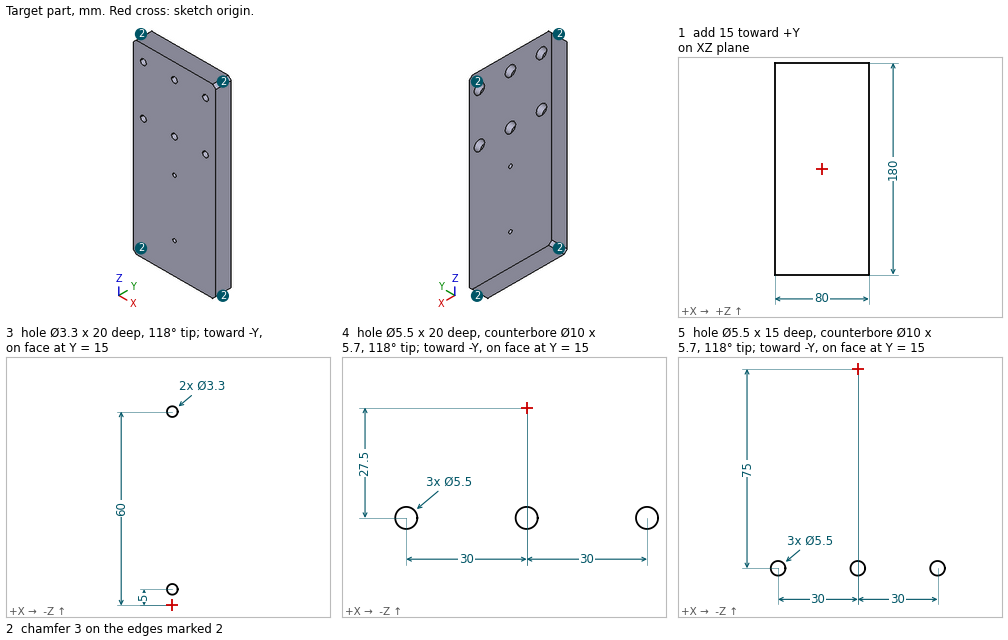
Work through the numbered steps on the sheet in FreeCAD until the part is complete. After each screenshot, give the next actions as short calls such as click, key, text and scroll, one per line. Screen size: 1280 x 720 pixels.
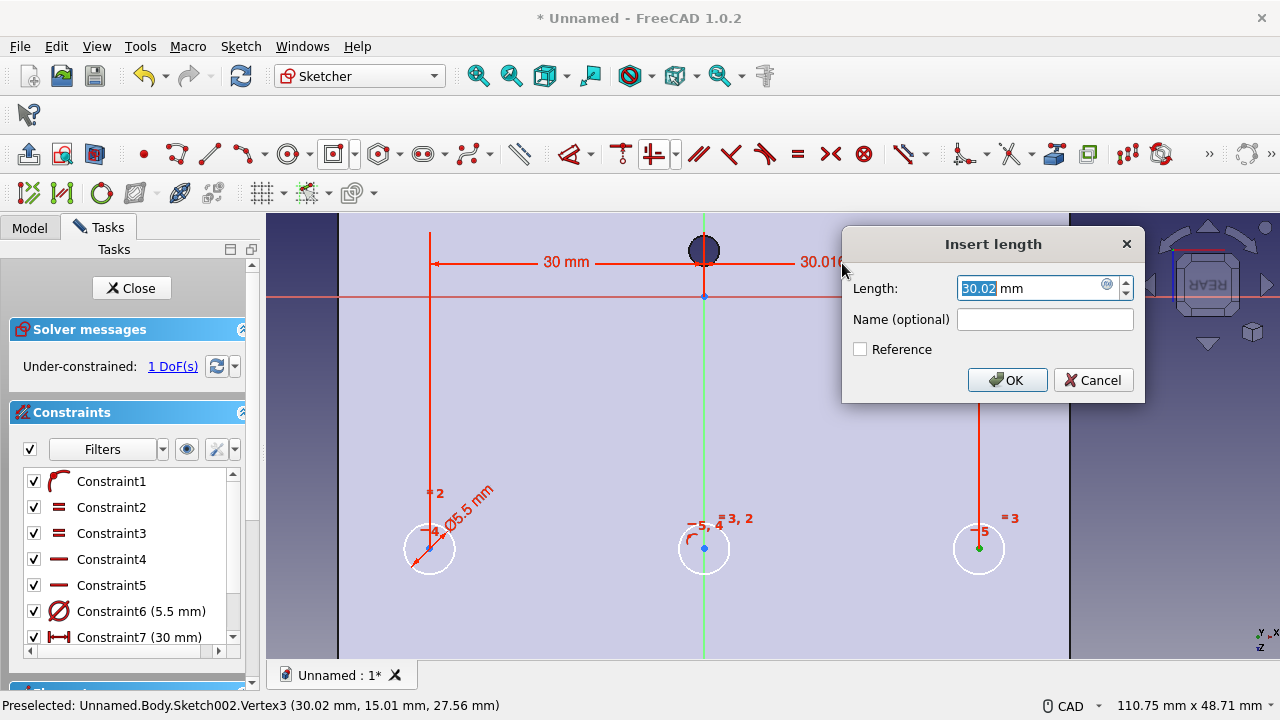
text(30)
key(Return)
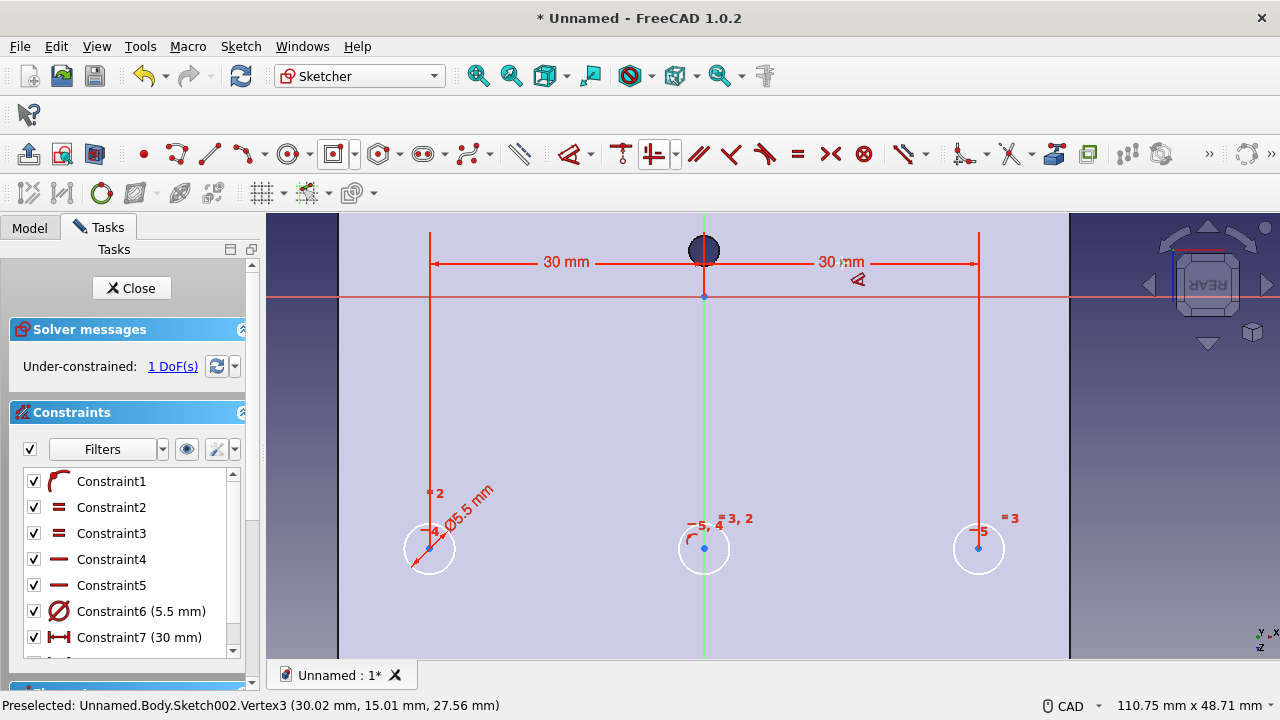
click(430, 549)
click(396, 423)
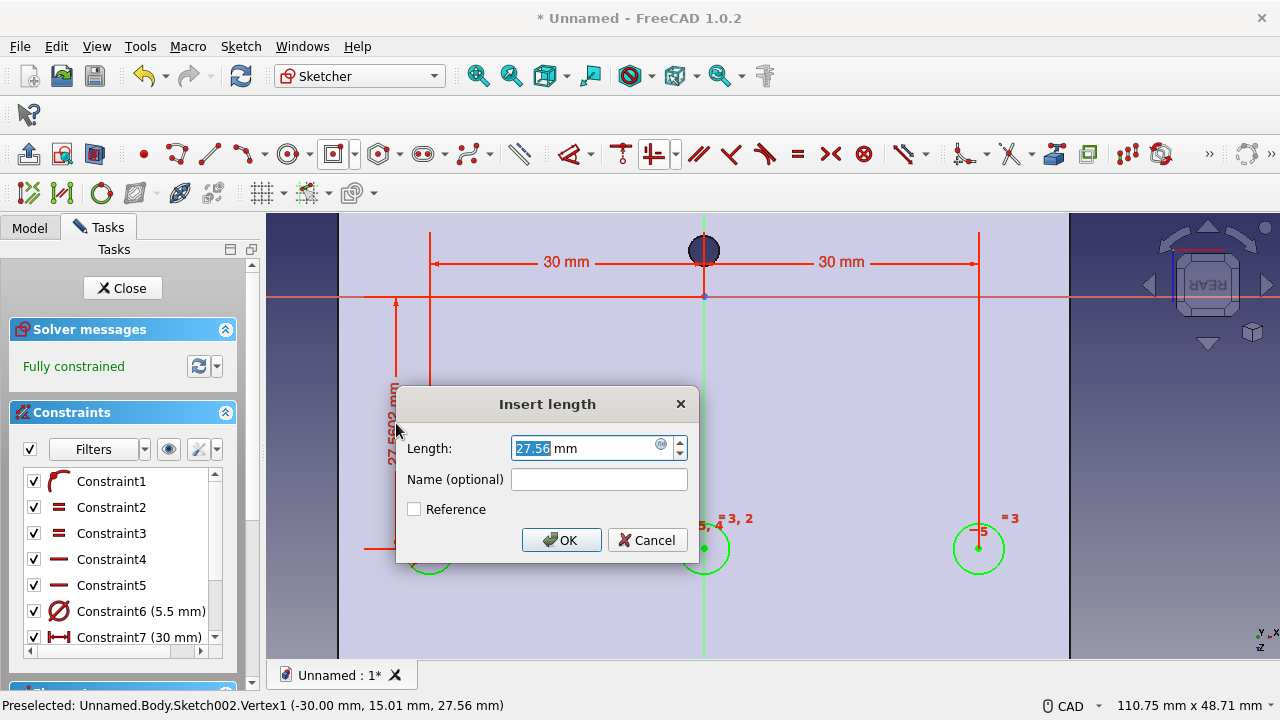
text(27.5)
key(Return)
key(Escape)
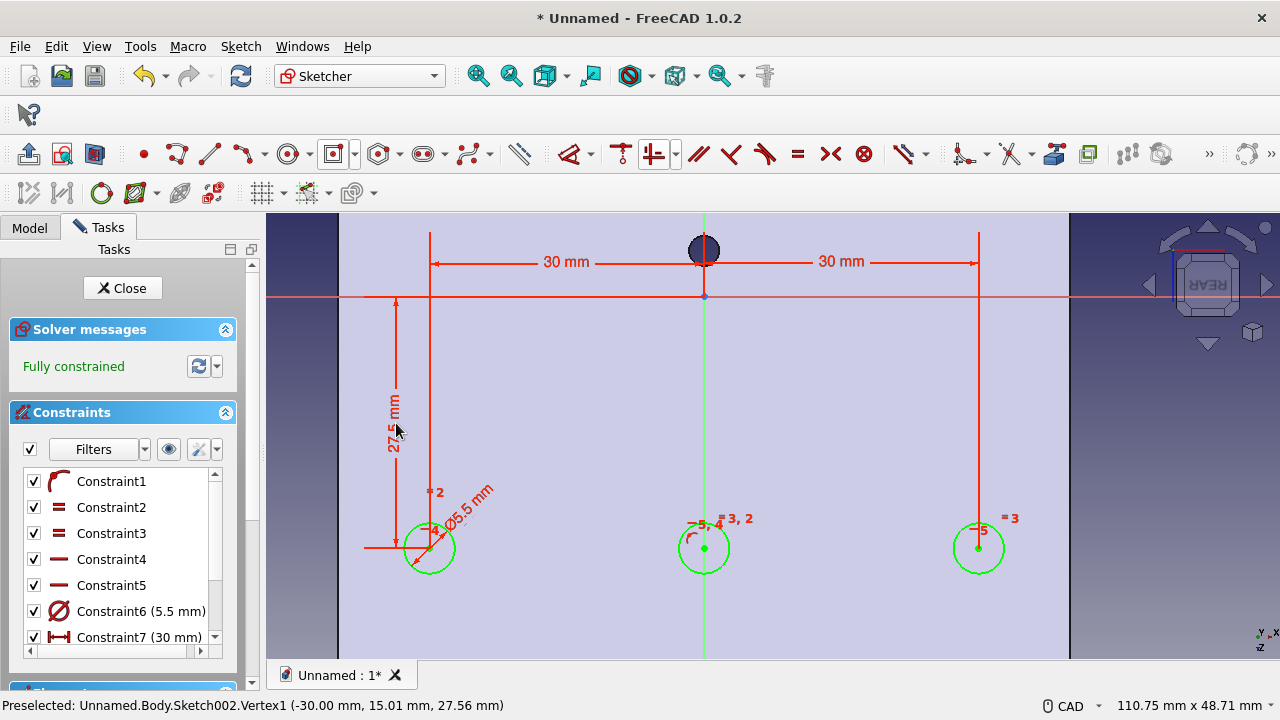
click(123, 288)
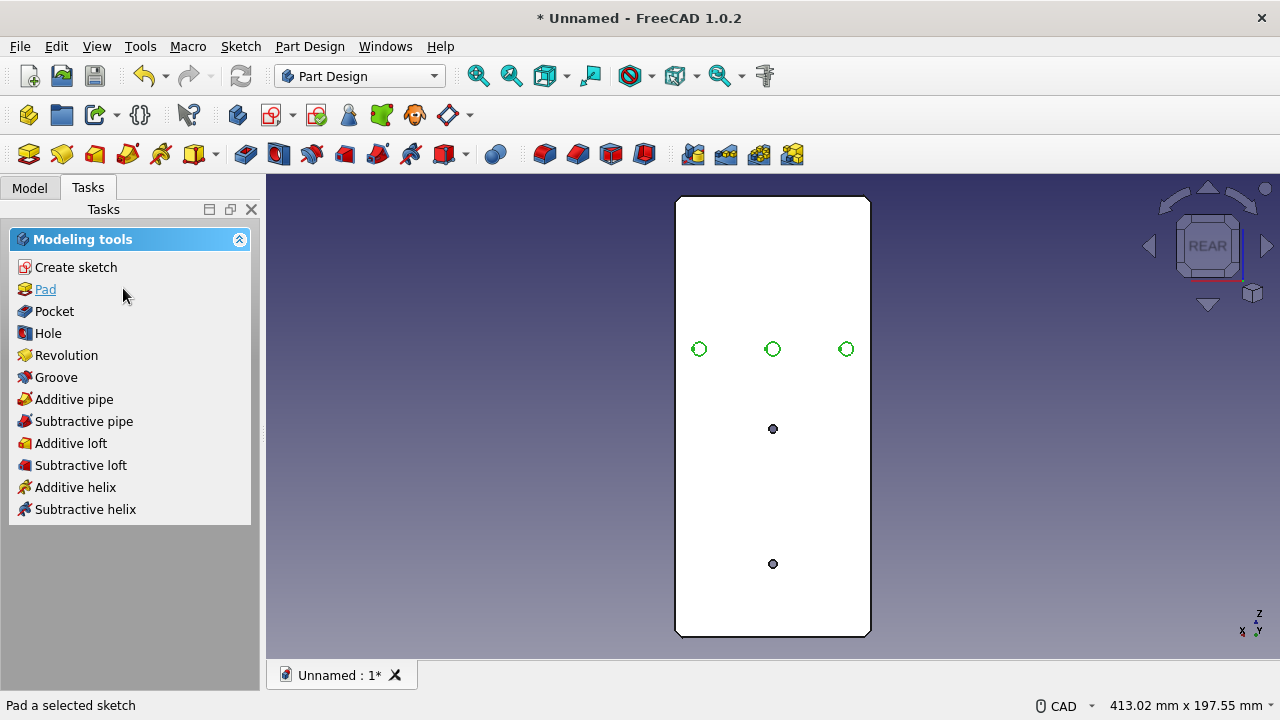
click(279, 154)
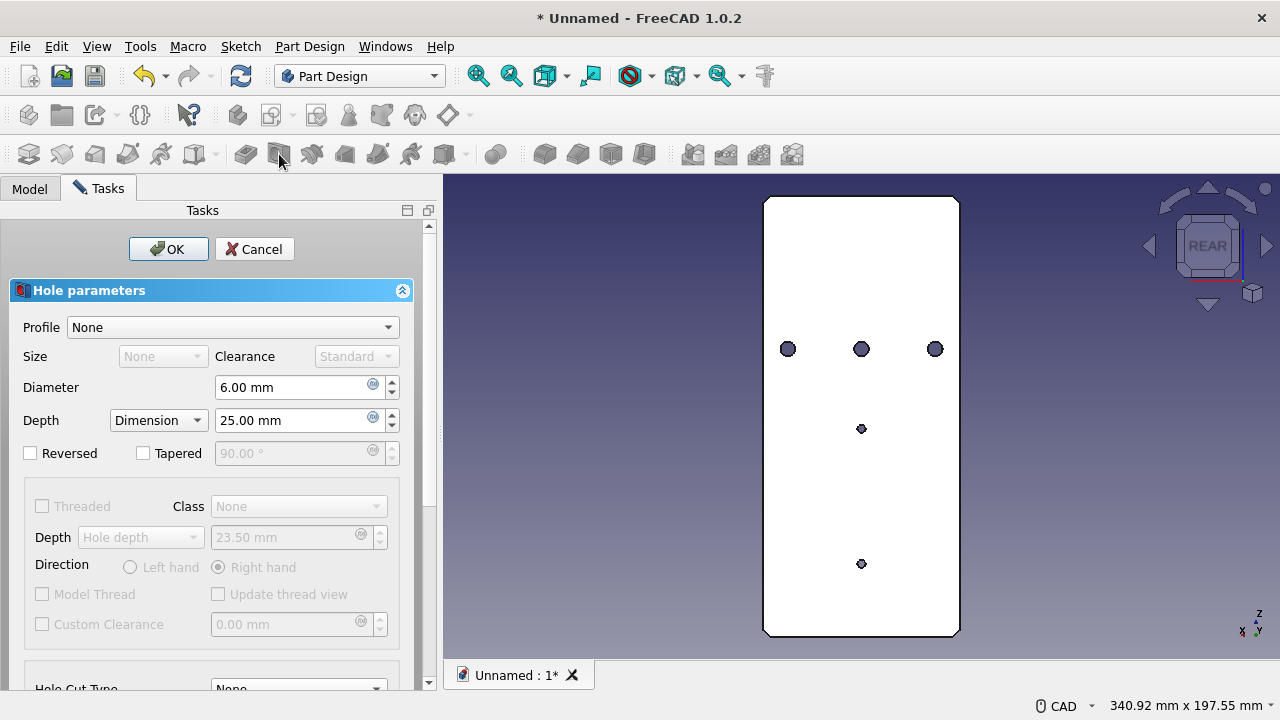
triple_click(300, 388)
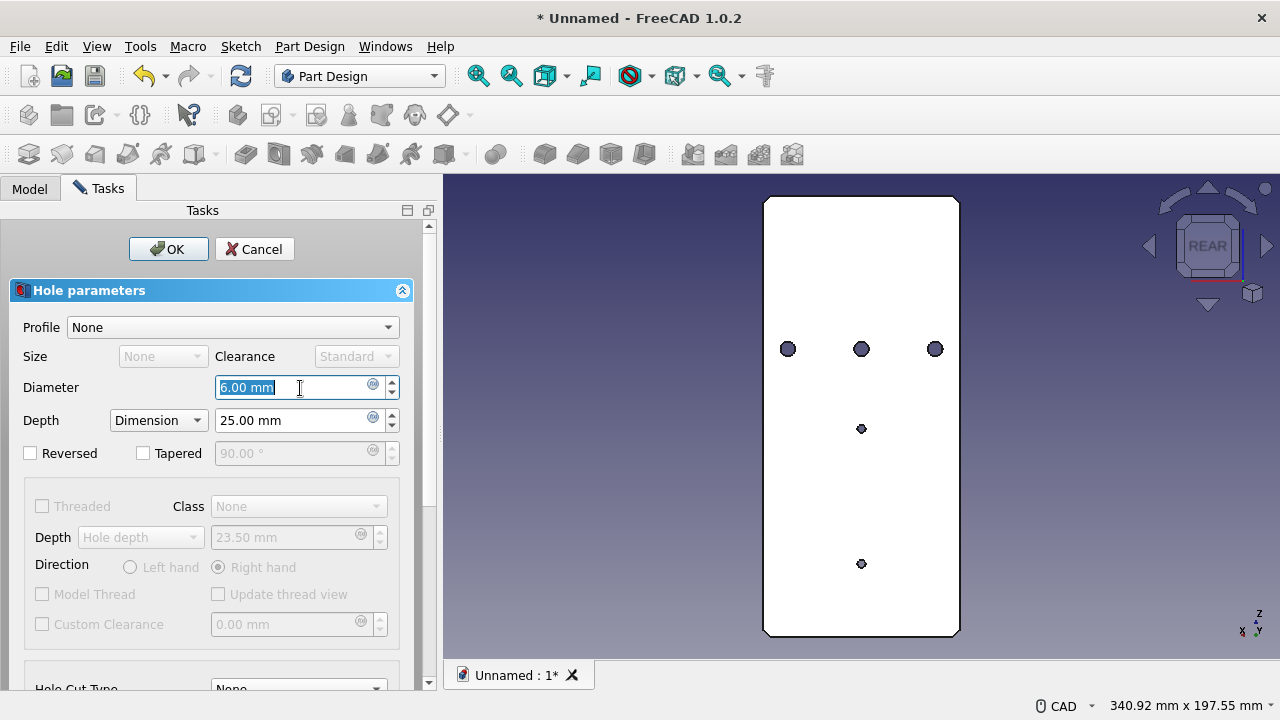
text(5.5)
key(Tab)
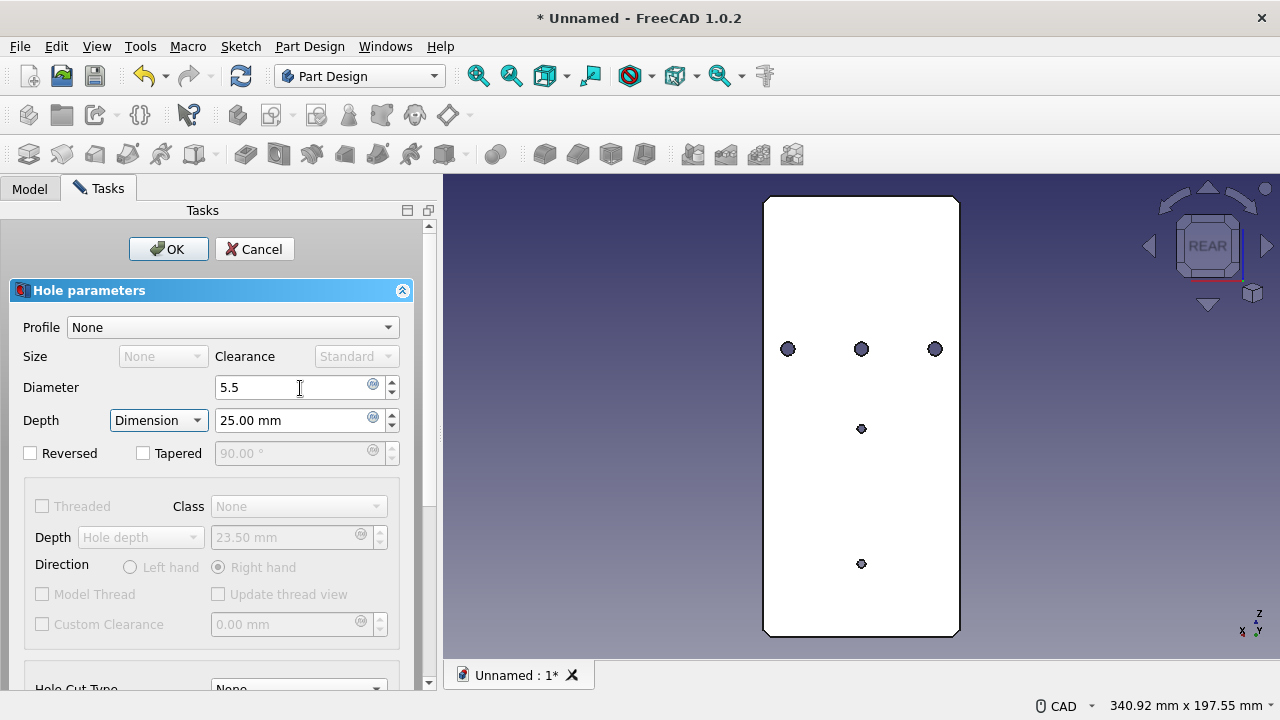
triple_click(300, 420)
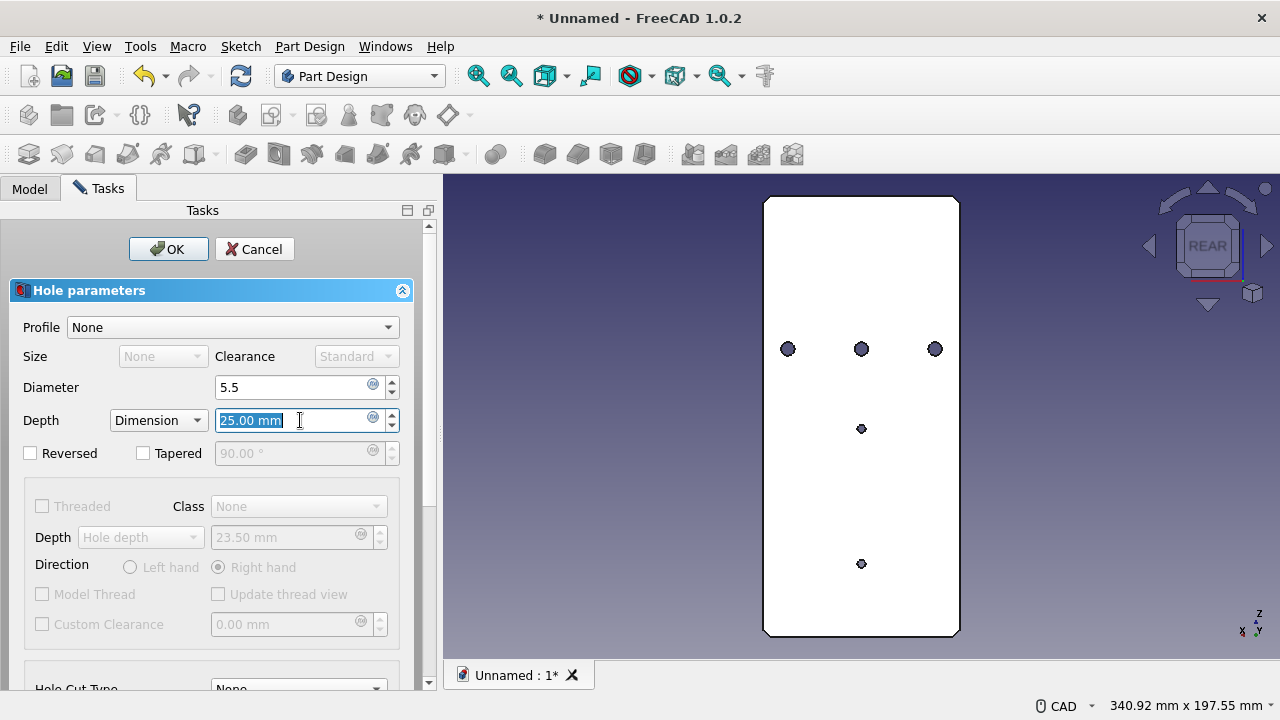
text(20)
key(Tab)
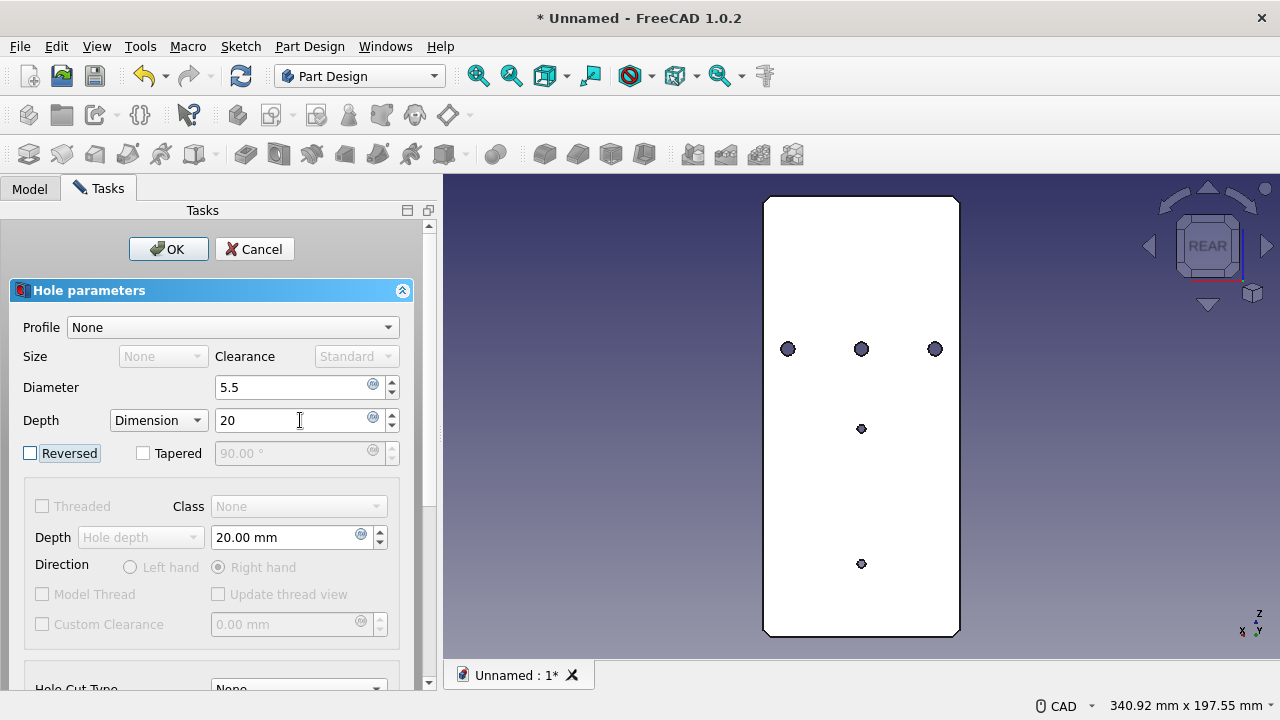
scroll(429, 455, down, 2)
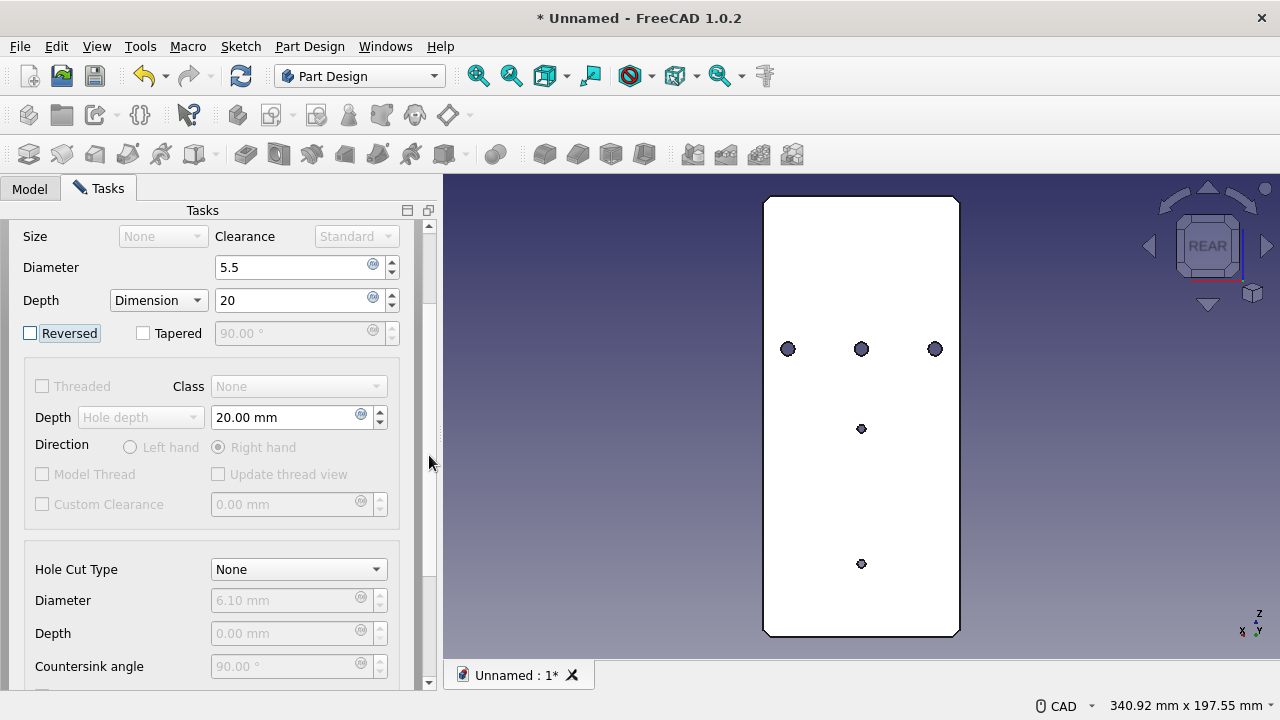
click(300, 570)